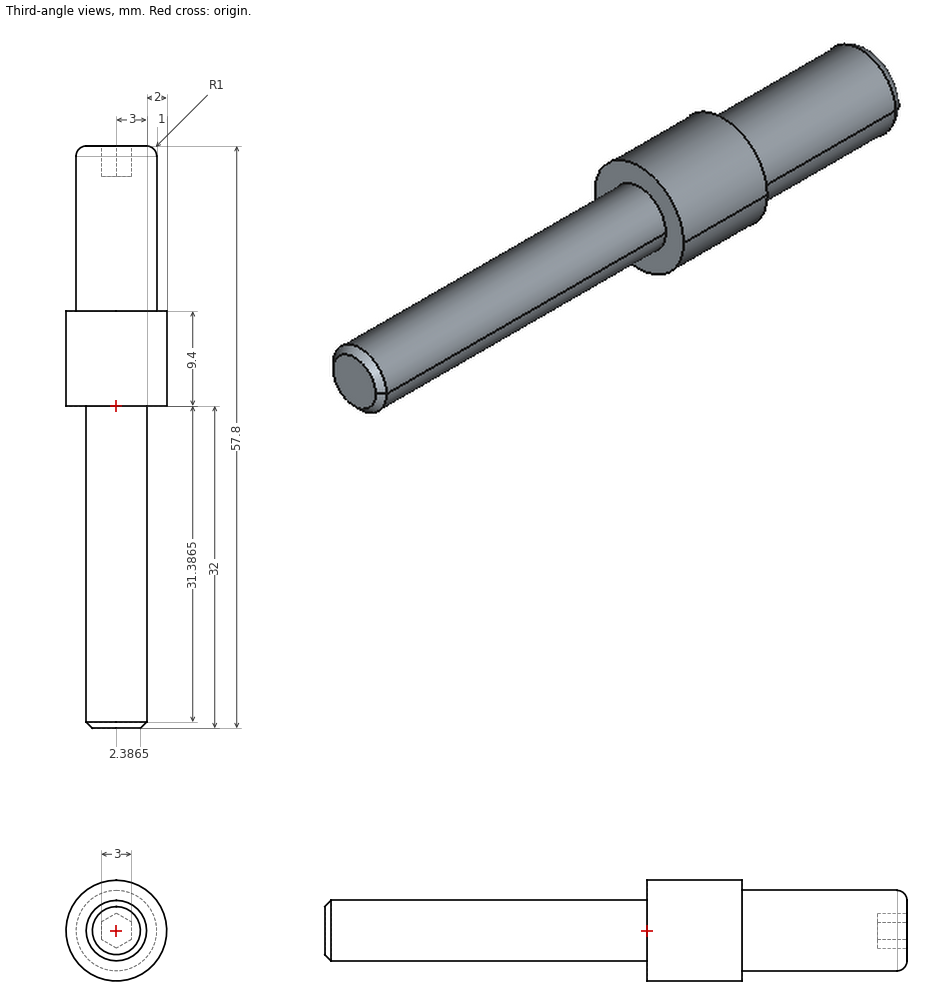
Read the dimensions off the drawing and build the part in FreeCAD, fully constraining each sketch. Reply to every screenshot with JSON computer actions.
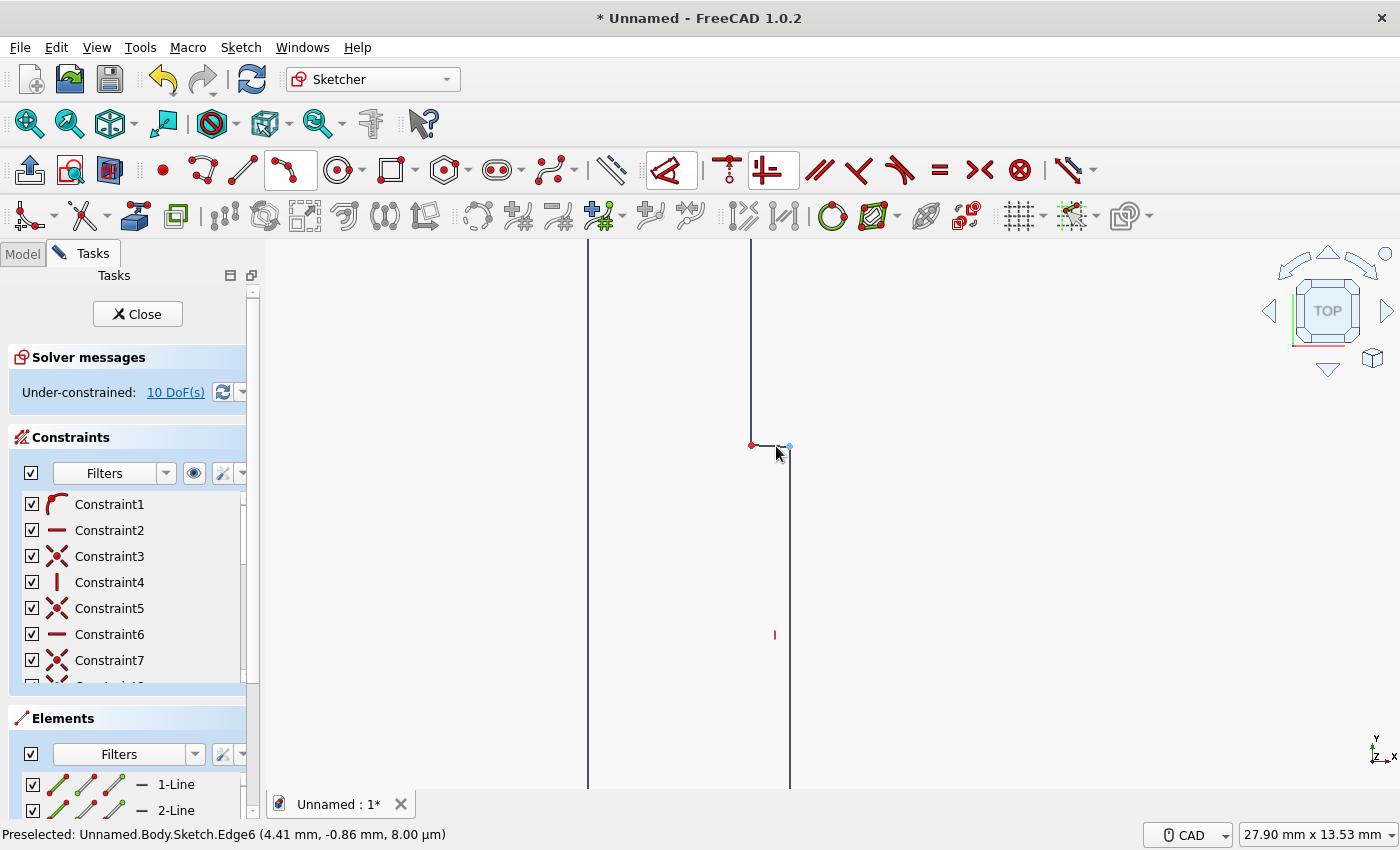
{"action": "left_click", "coordinate": [774, 446]}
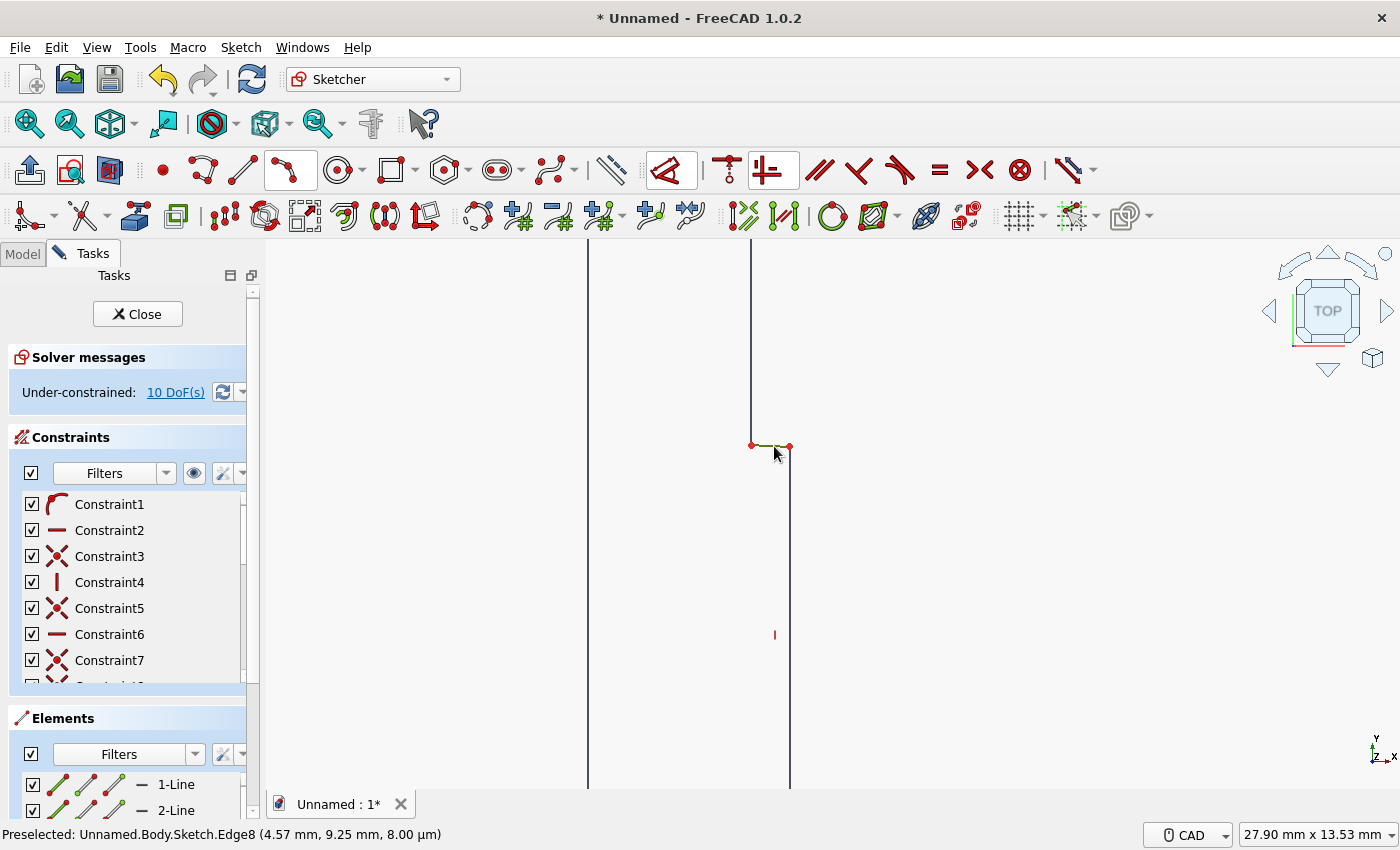
{"action": "left_click", "coordinate": [794, 170]}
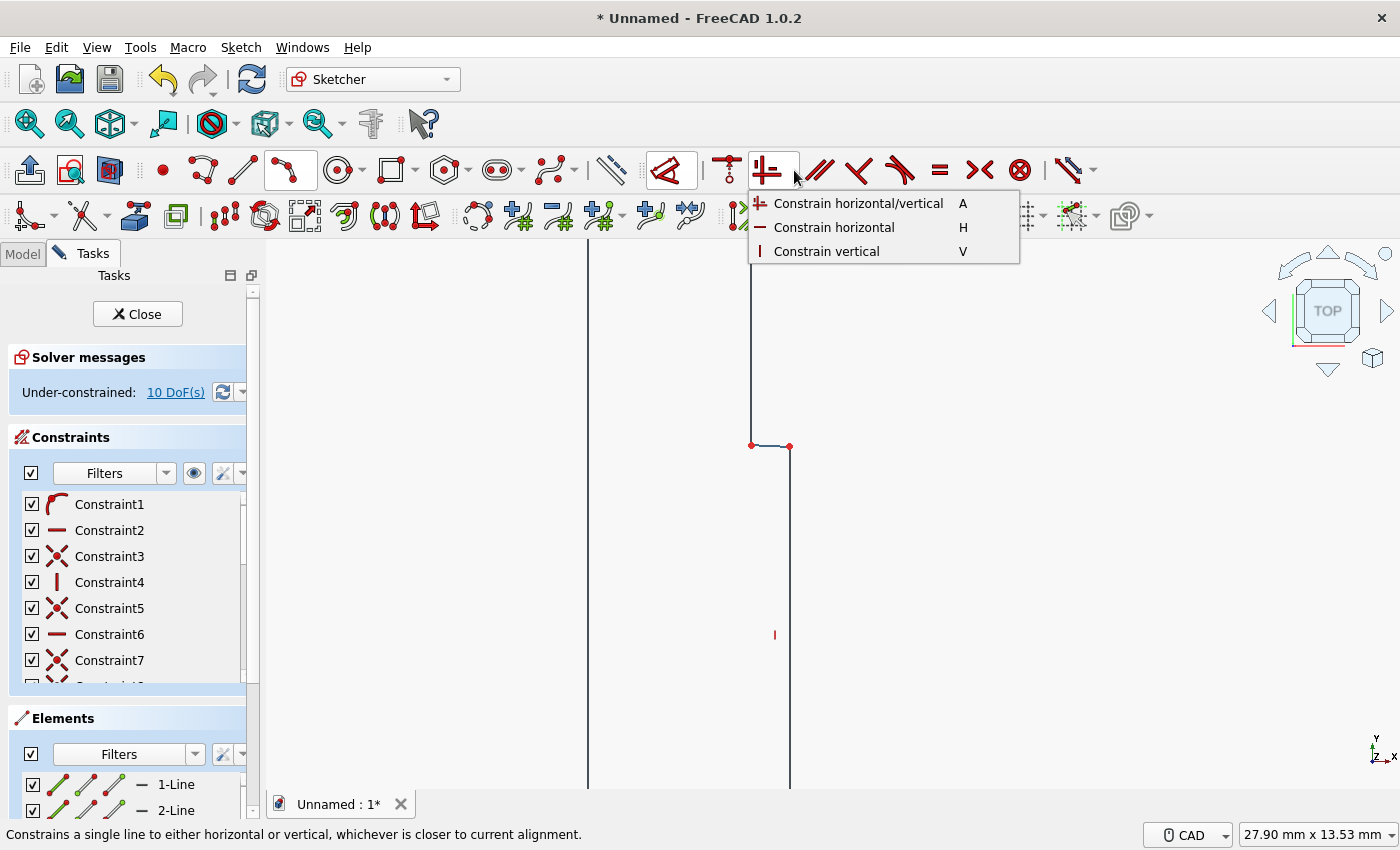
{"action": "left_click", "coordinate": [884, 227]}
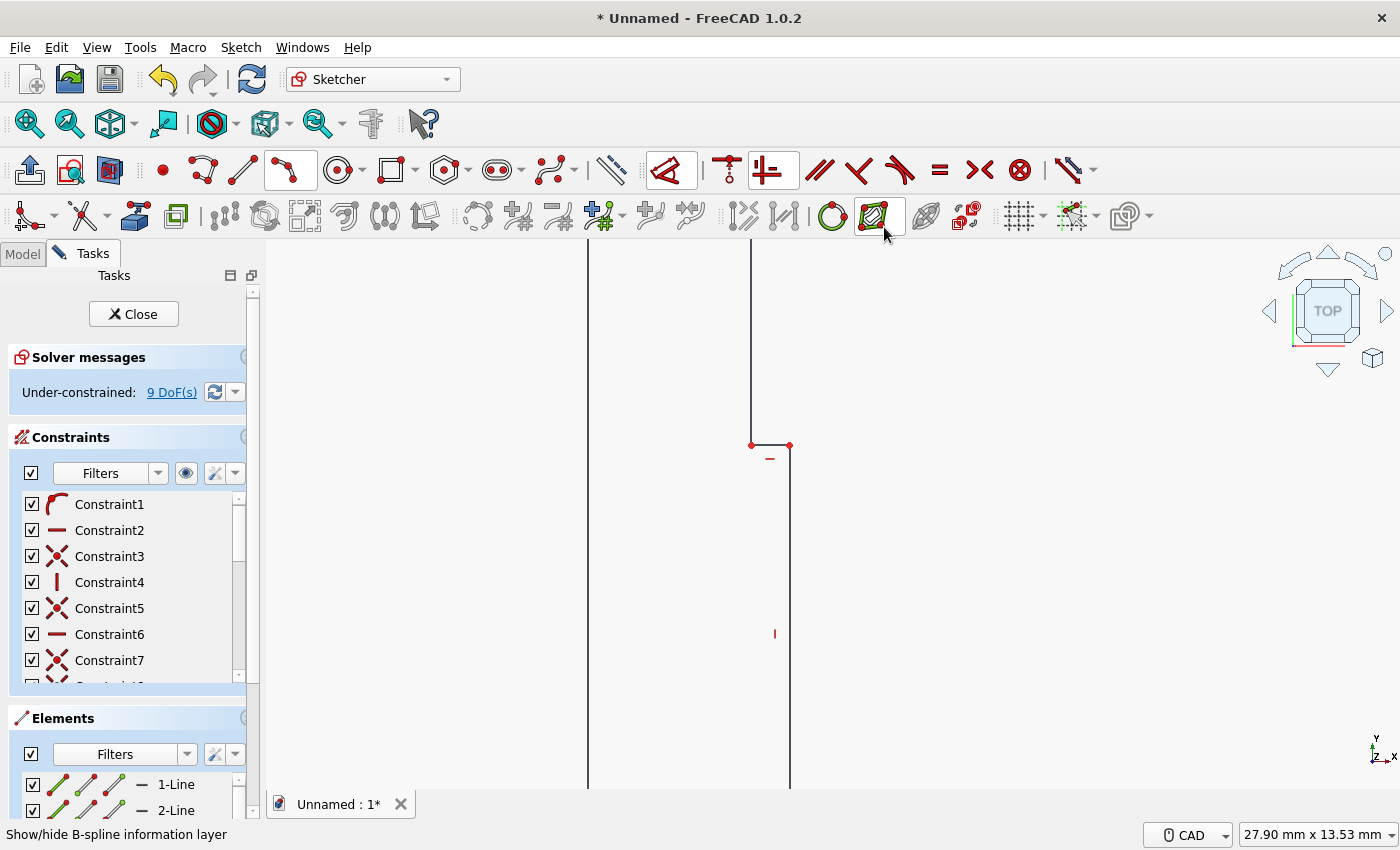
{"action": "left_click", "coordinate": [666, 170]}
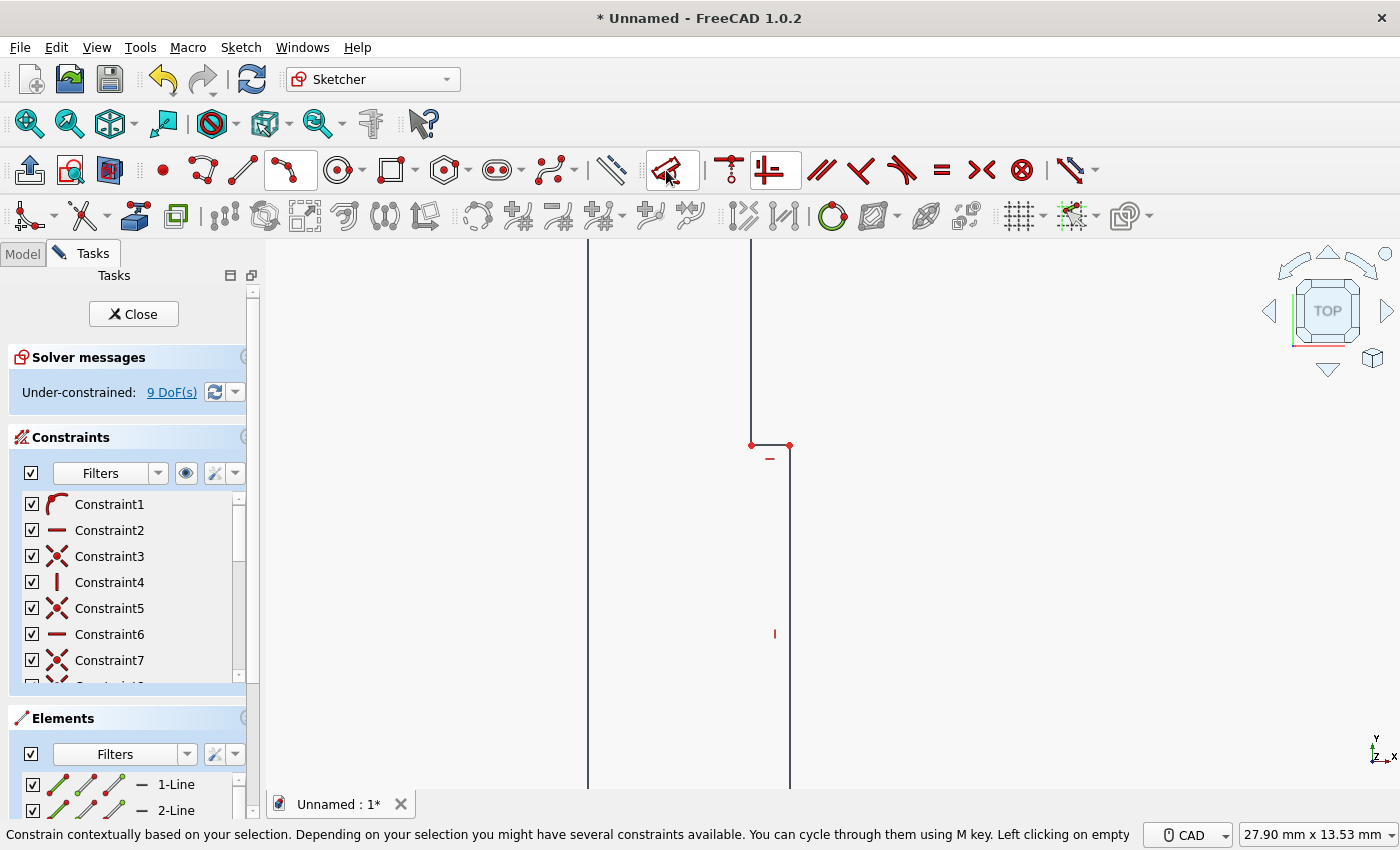
{"action": "scroll", "coordinate": [776, 446], "scroll_direction": "down", "scroll_amount": 10}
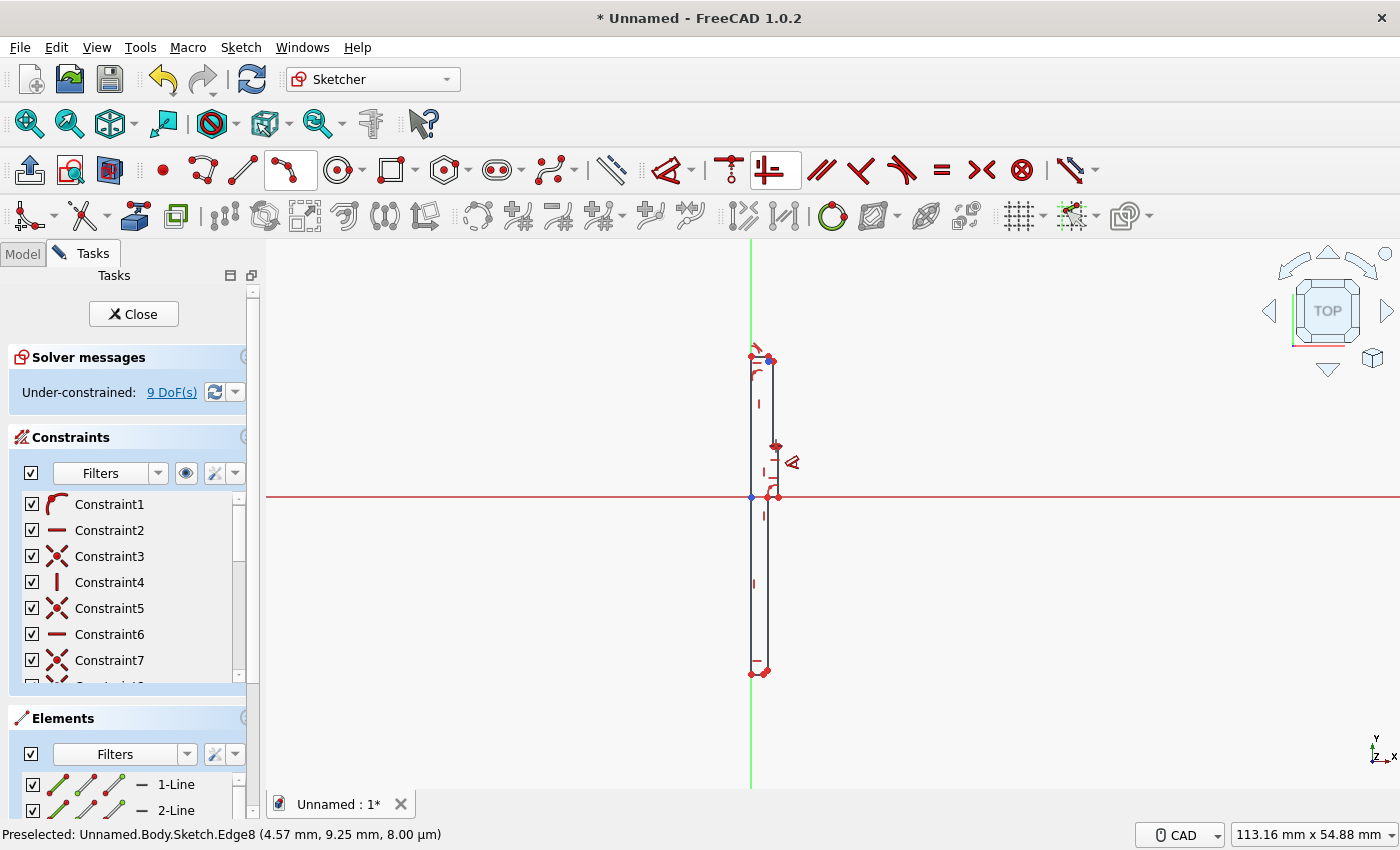
{"action": "scroll", "coordinate": [773, 359], "scroll_direction": "up", "scroll_amount": 10}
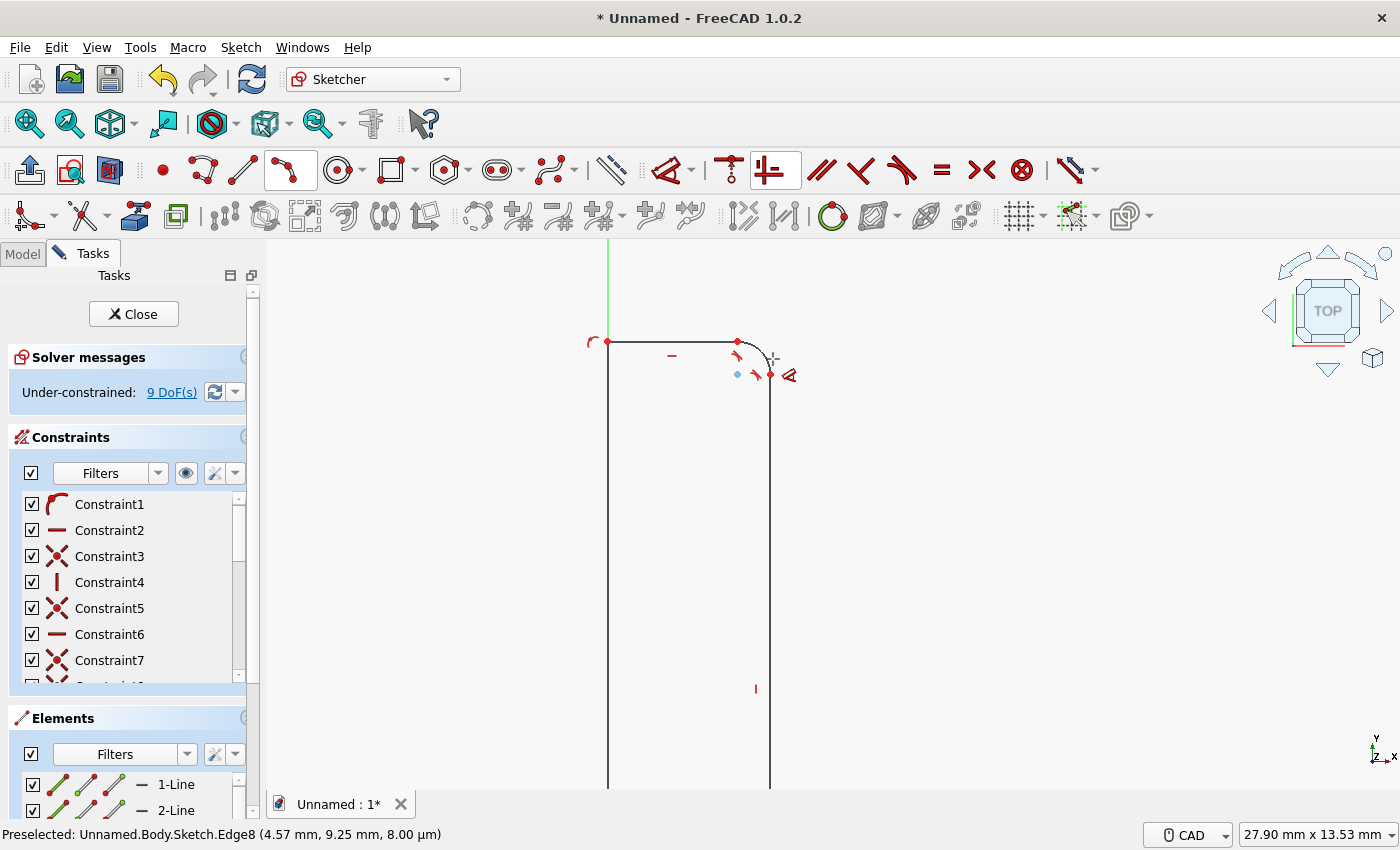
{"action": "left_click", "coordinate": [767, 360]}
{"action": "left_click", "coordinate": [796, 346]}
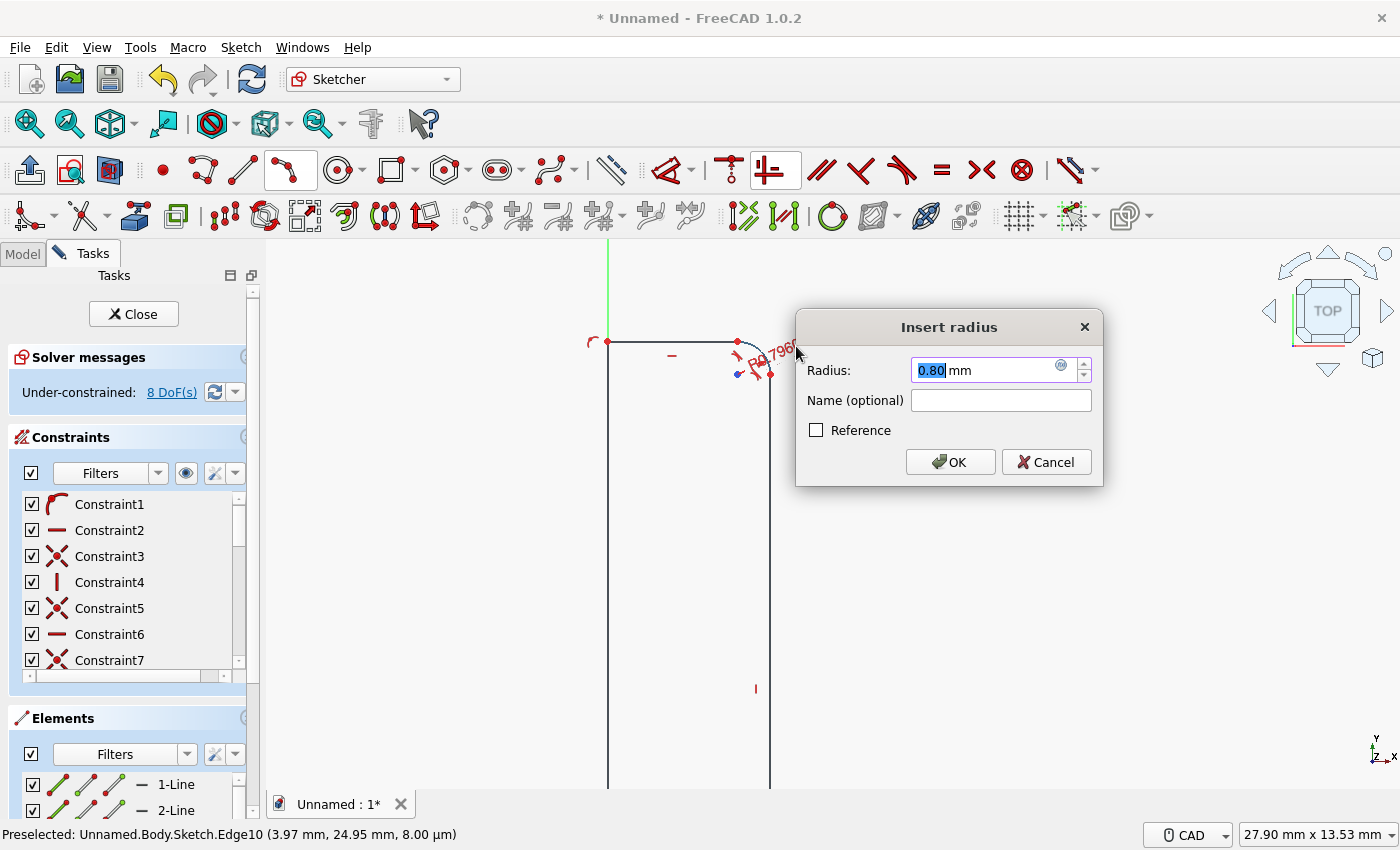
{"action": "type", "text": "1"}
{"action": "key", "text": "Return"}